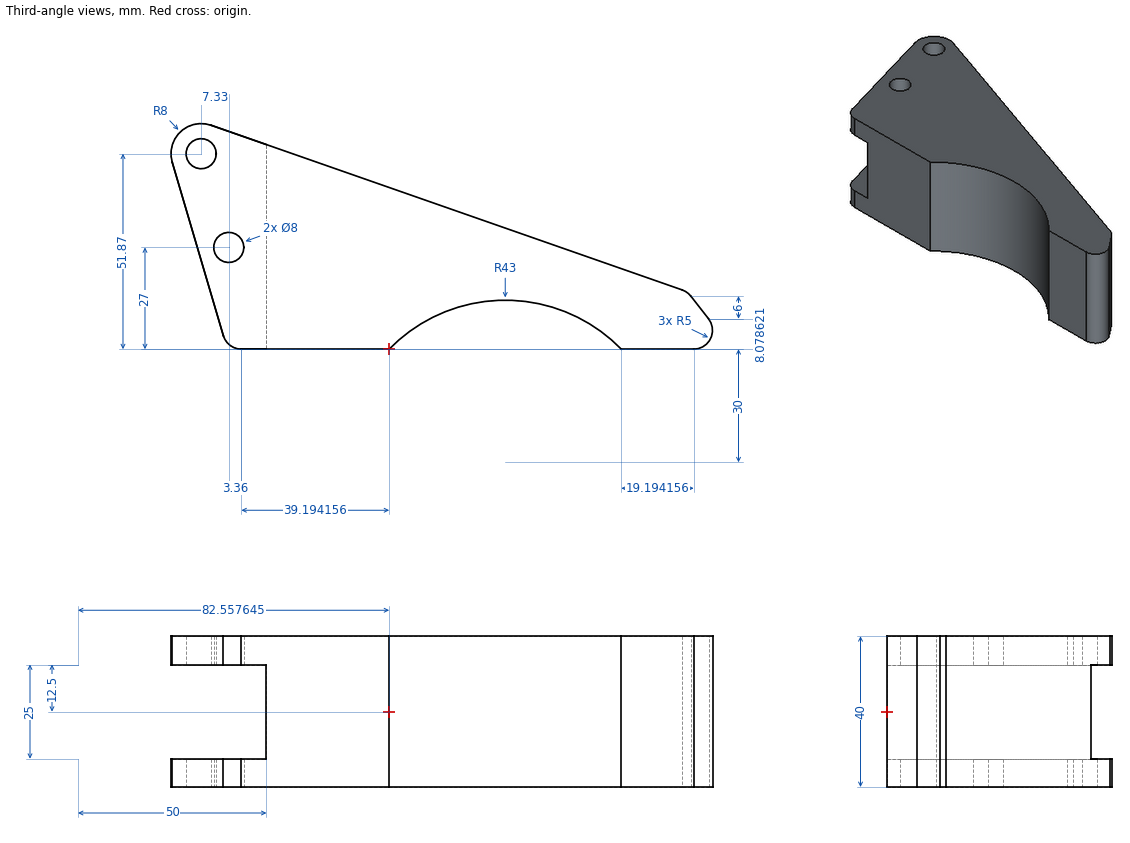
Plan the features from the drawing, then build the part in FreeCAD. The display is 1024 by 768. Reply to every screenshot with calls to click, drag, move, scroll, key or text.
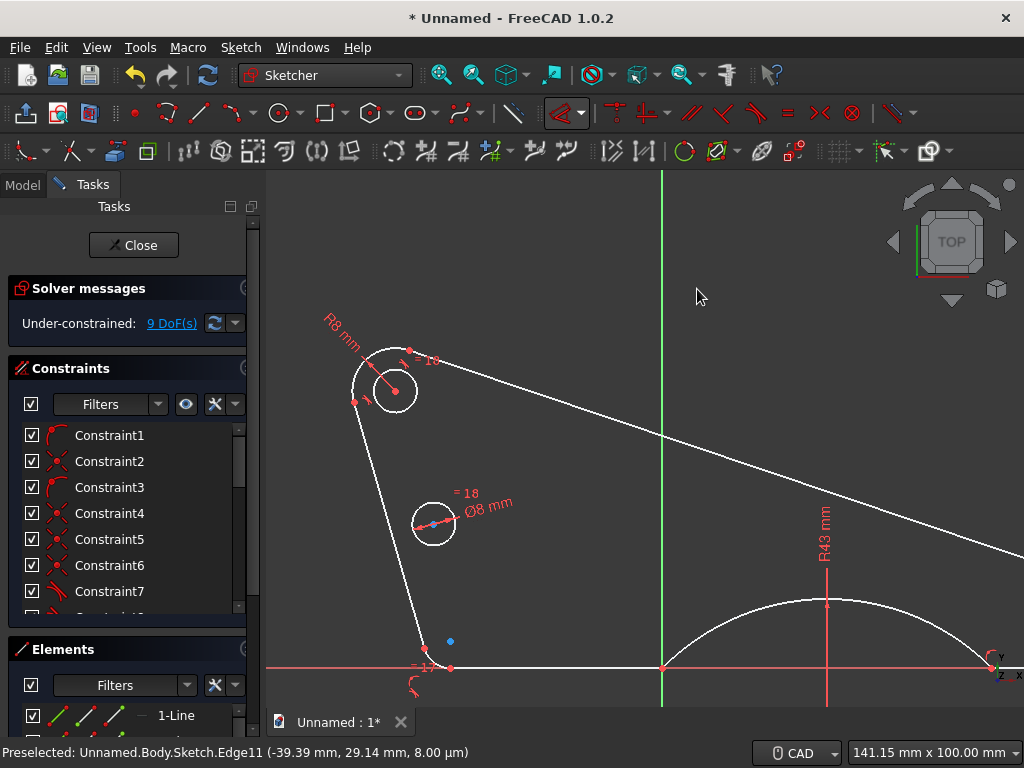
scroll(382, 353, down, 3)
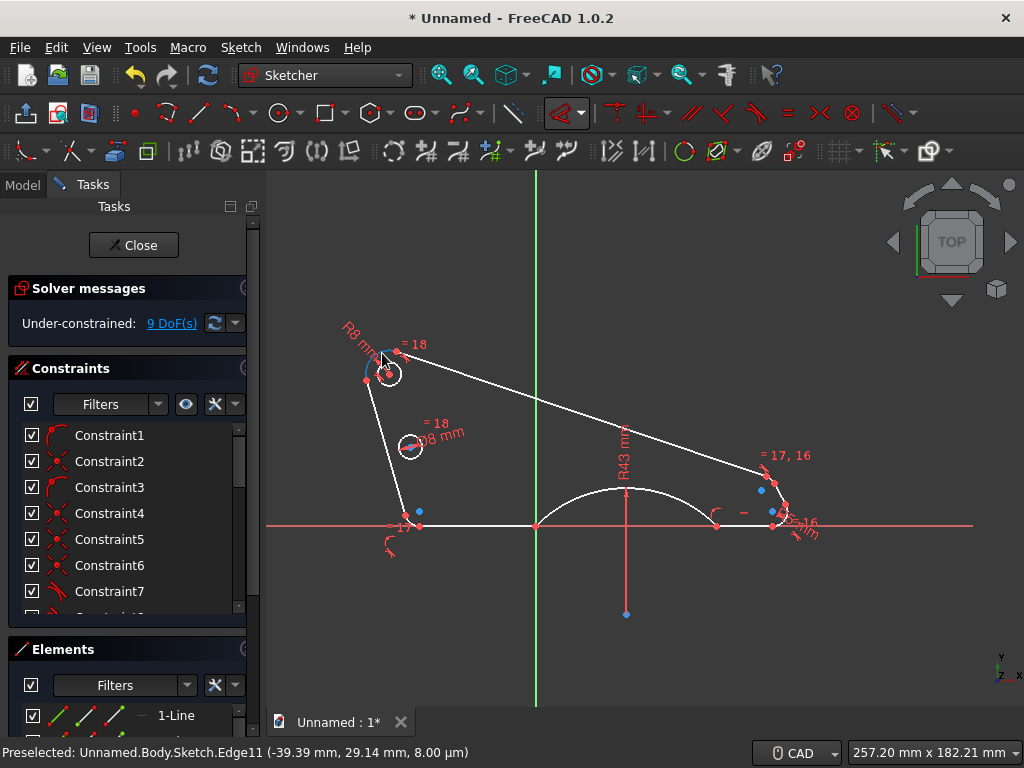
scroll(782, 498, up, 5)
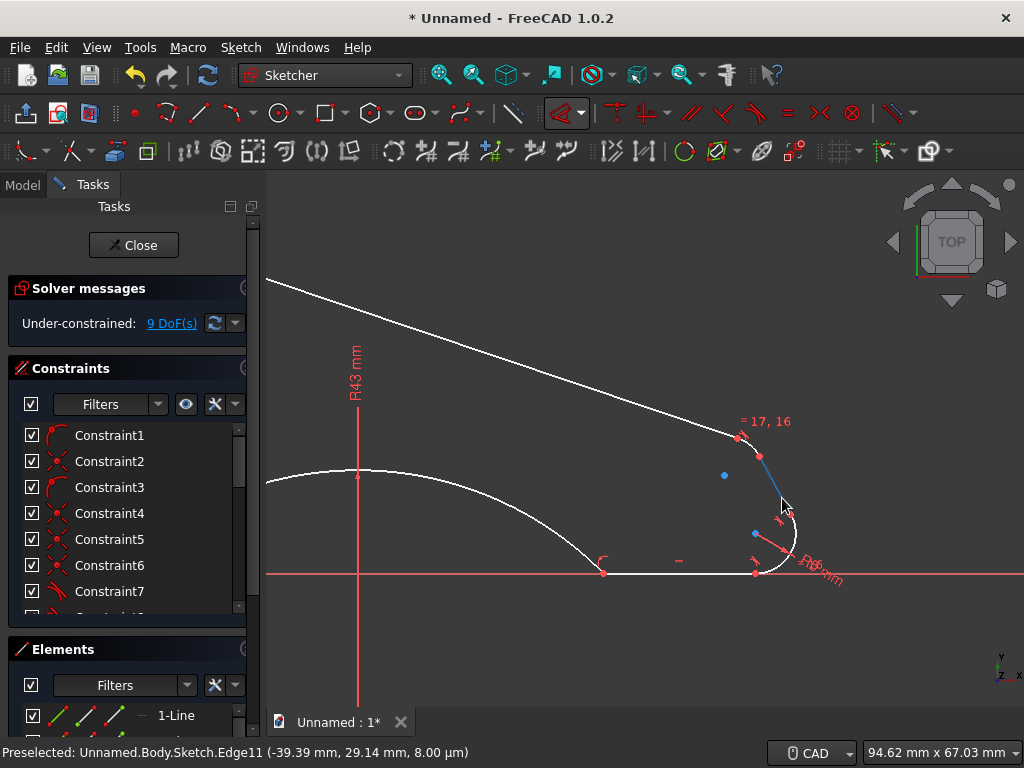
click(782, 497)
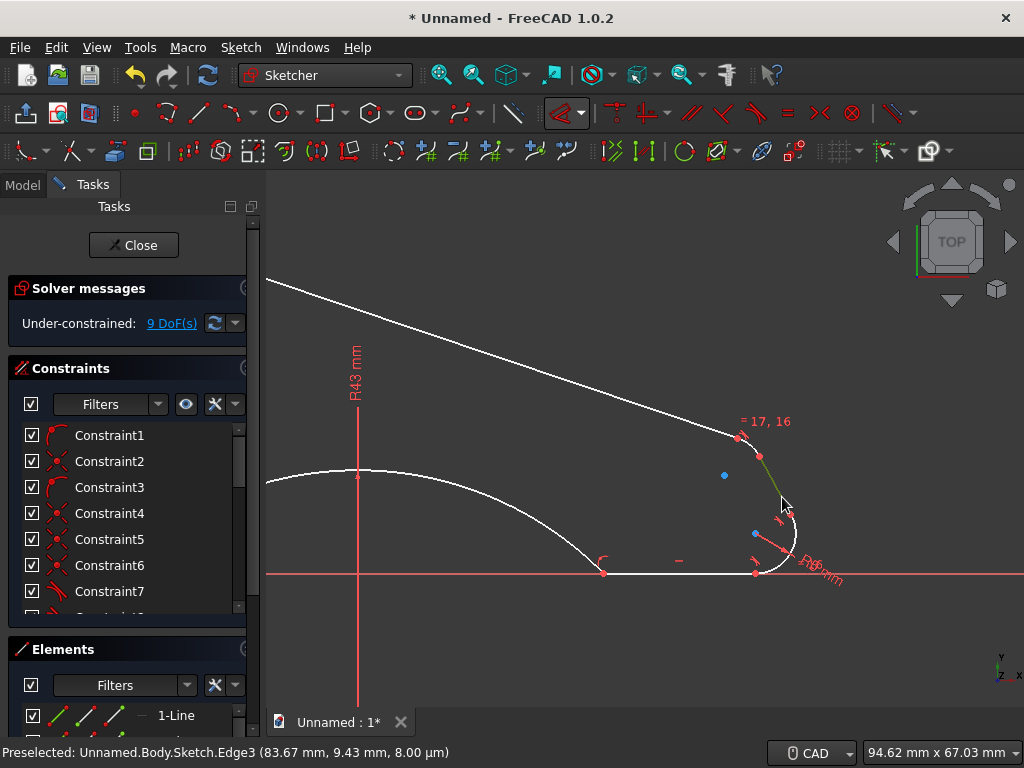
key(i)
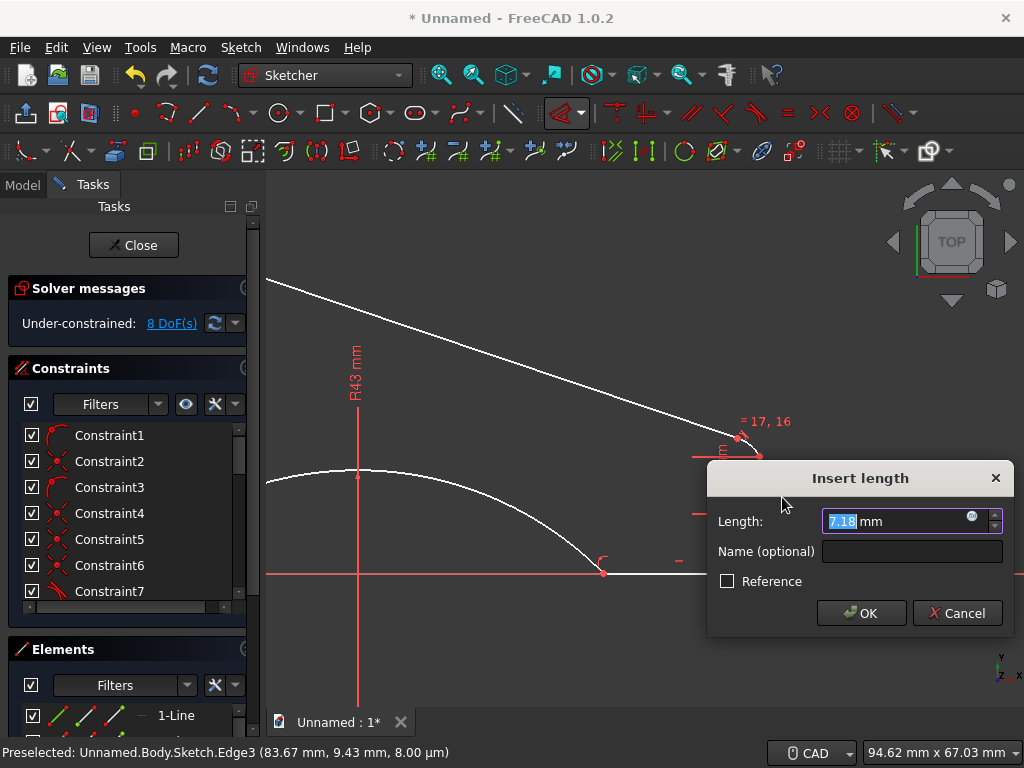
text(6)
key(Return)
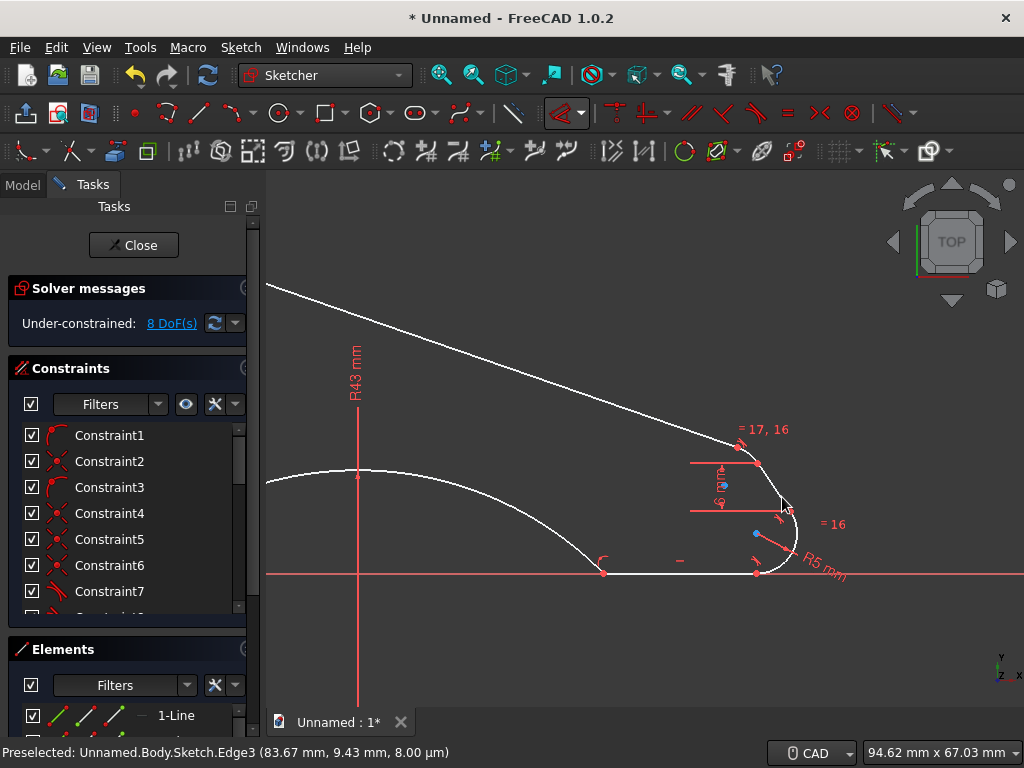
scroll(782, 498, down, 5)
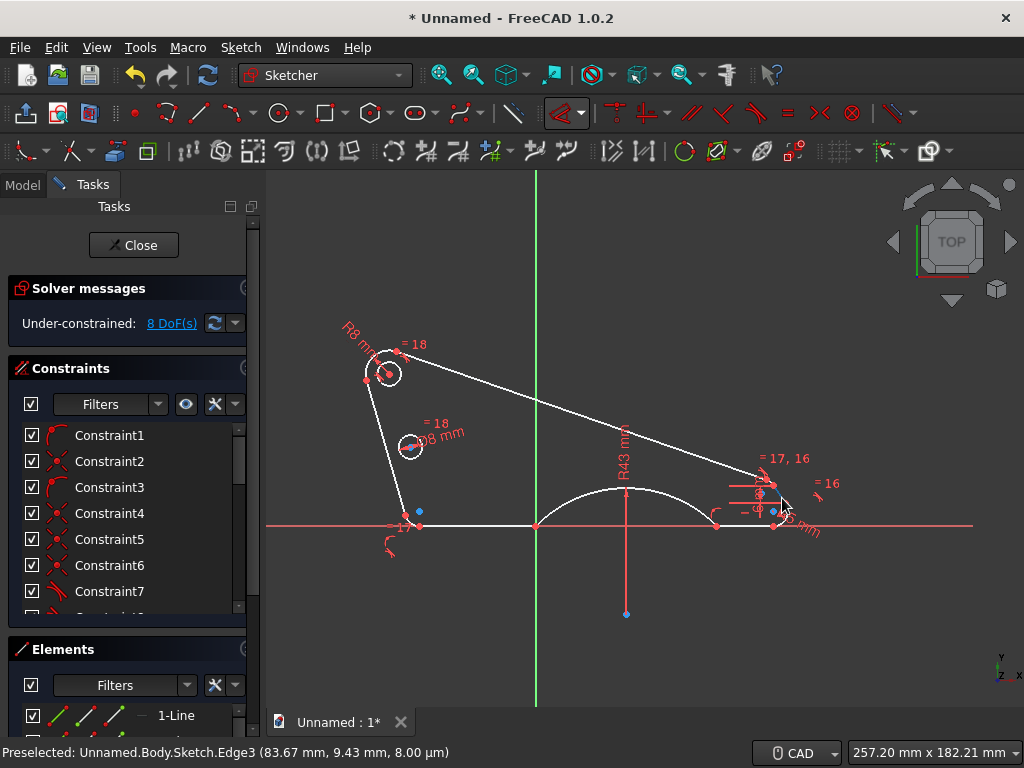
click(411, 447)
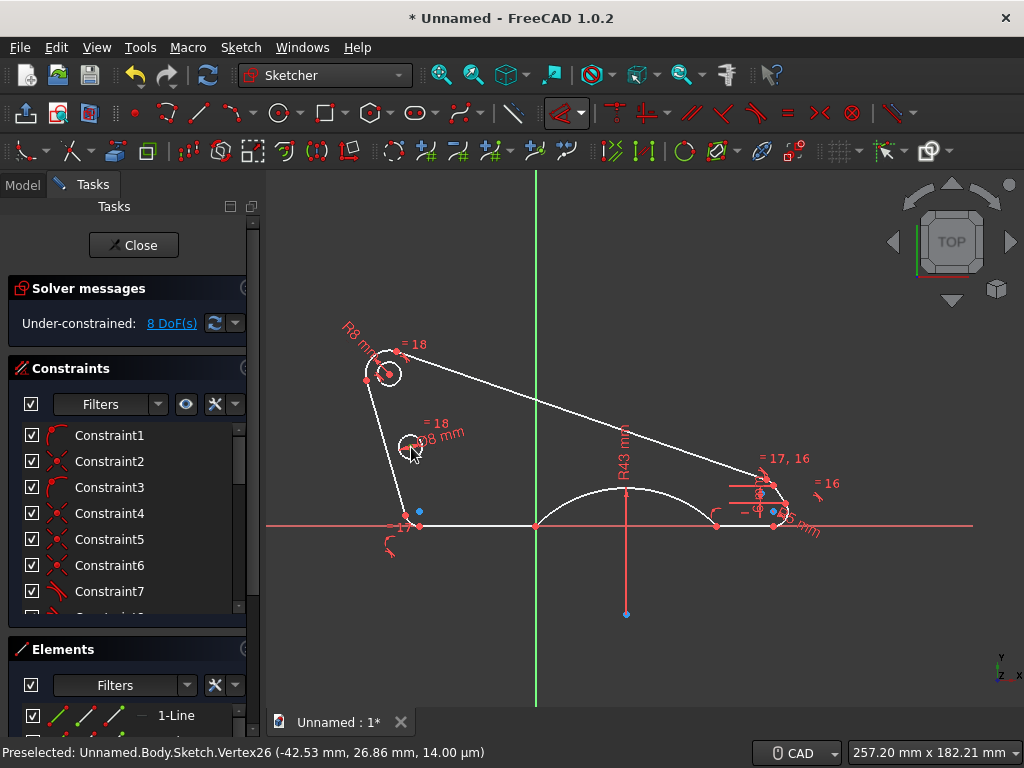
key(i)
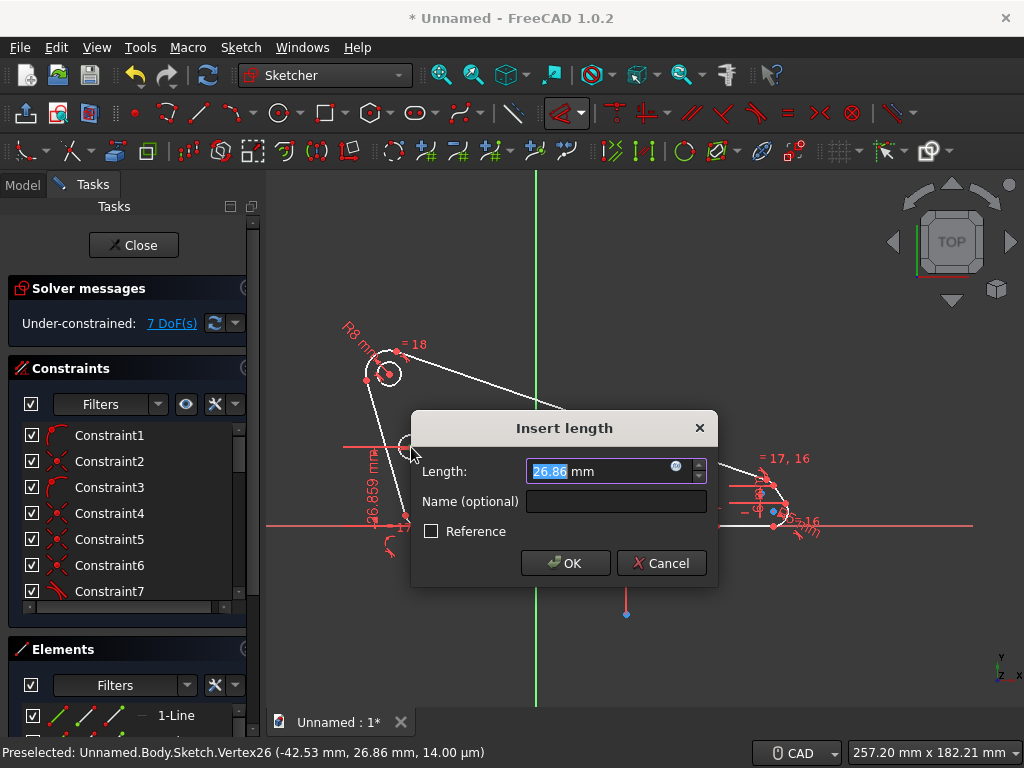
text(27)
key(Return)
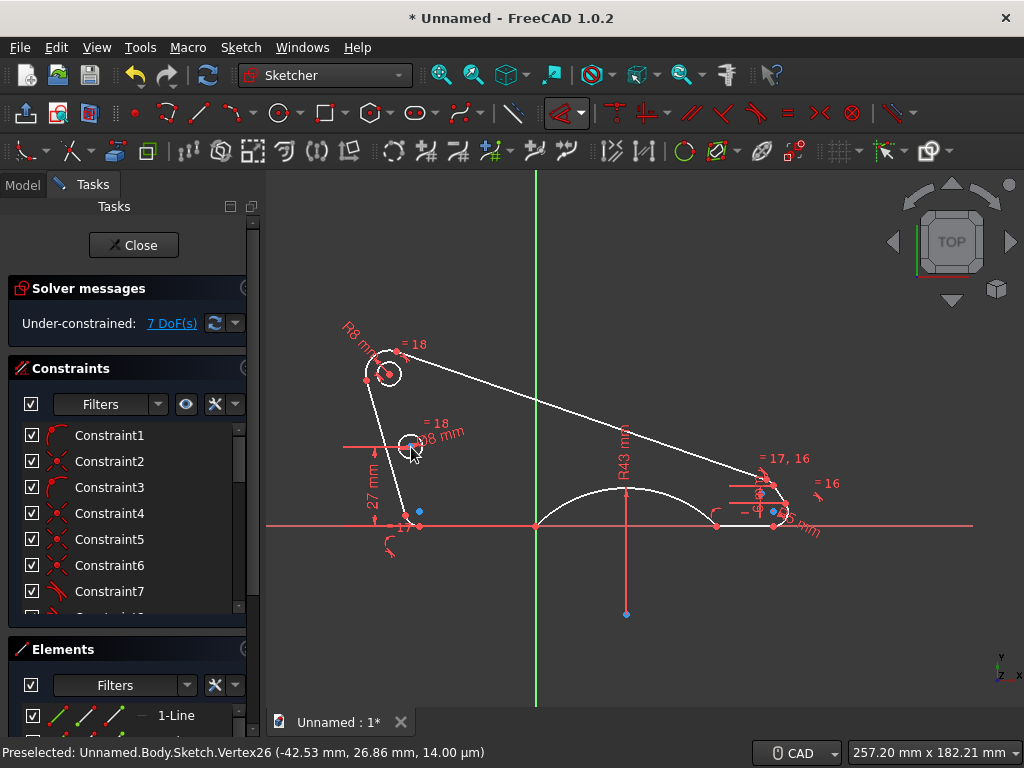
click(626, 615)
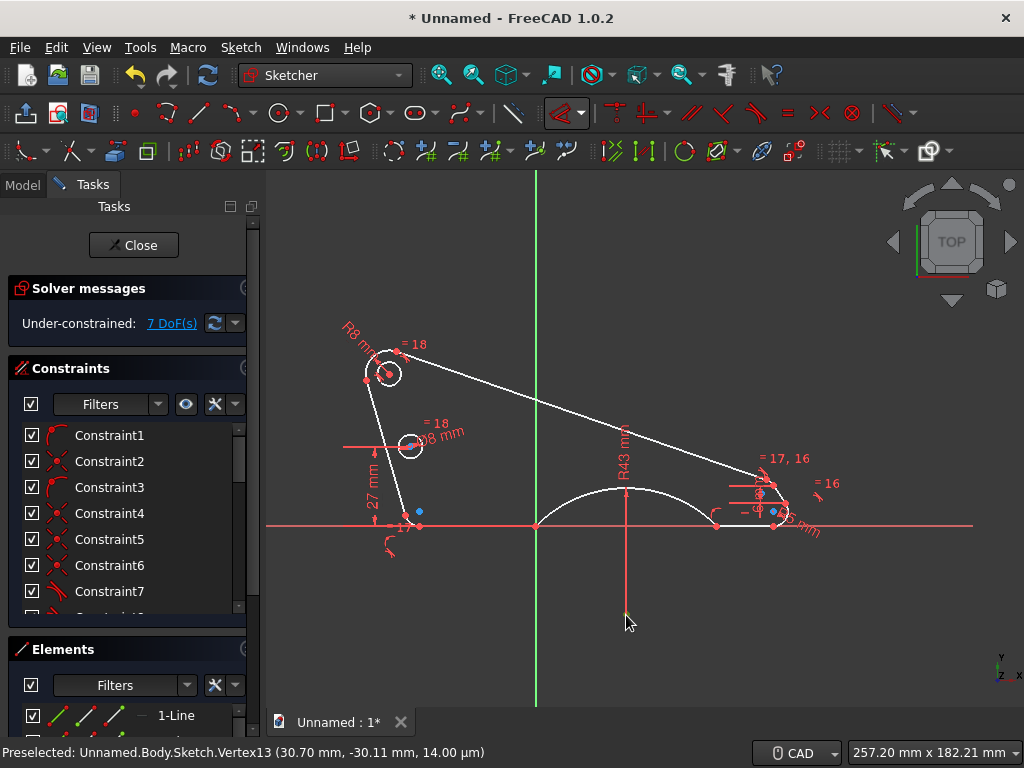
click(584, 114)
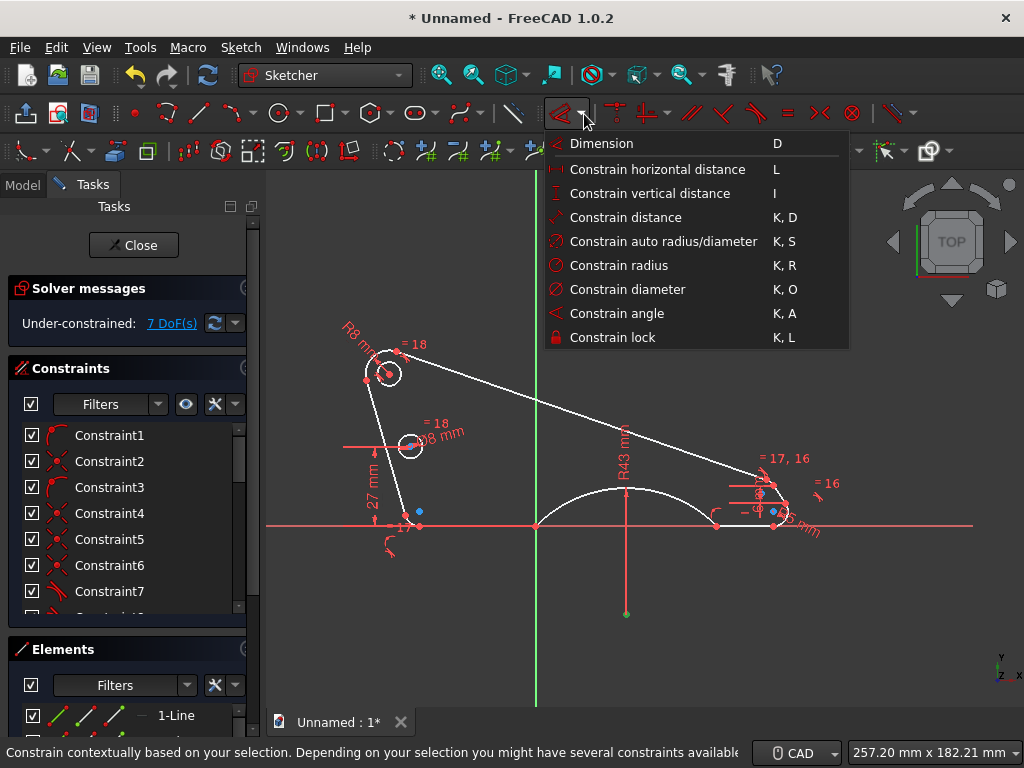
click(697, 193)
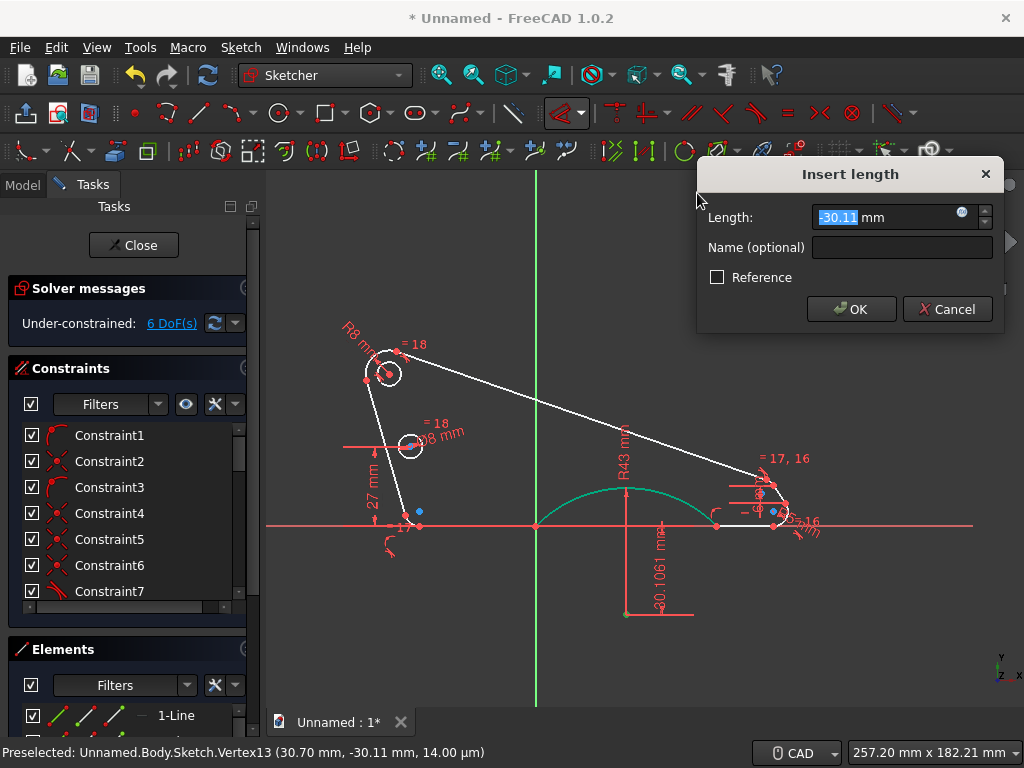
text(-30)
key(Return)